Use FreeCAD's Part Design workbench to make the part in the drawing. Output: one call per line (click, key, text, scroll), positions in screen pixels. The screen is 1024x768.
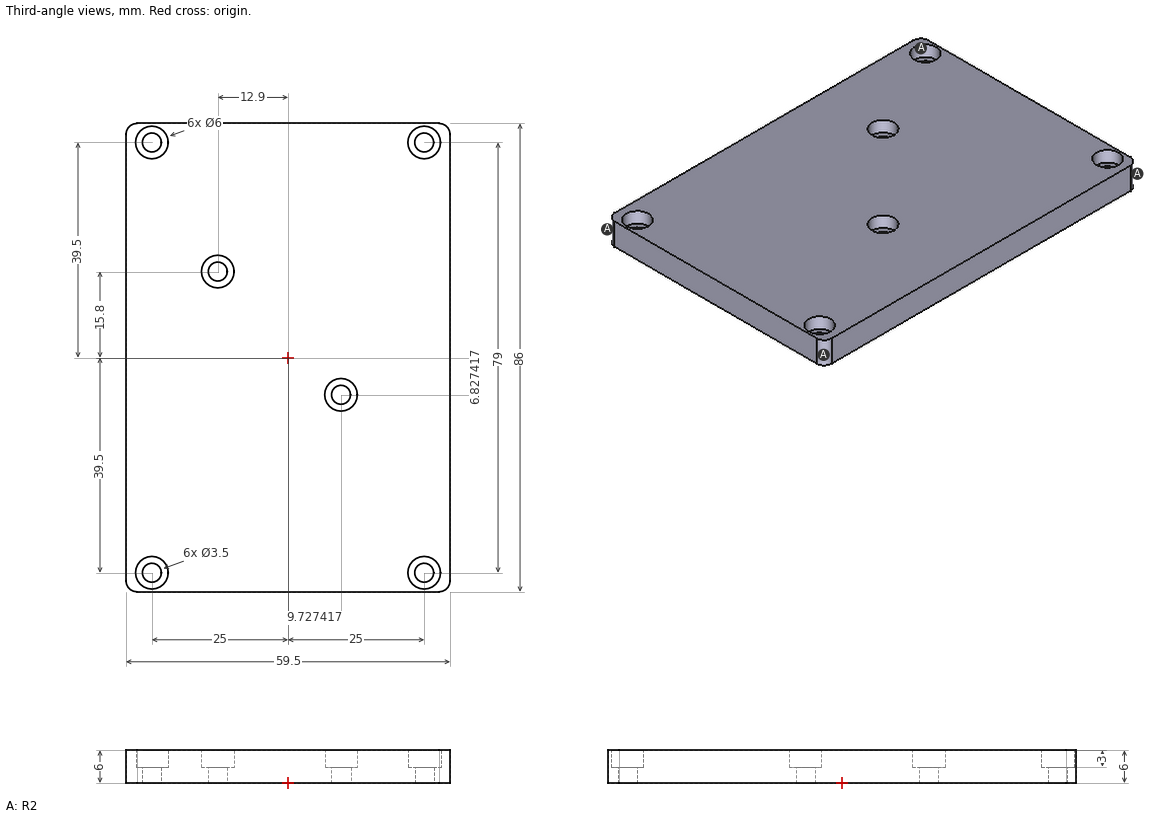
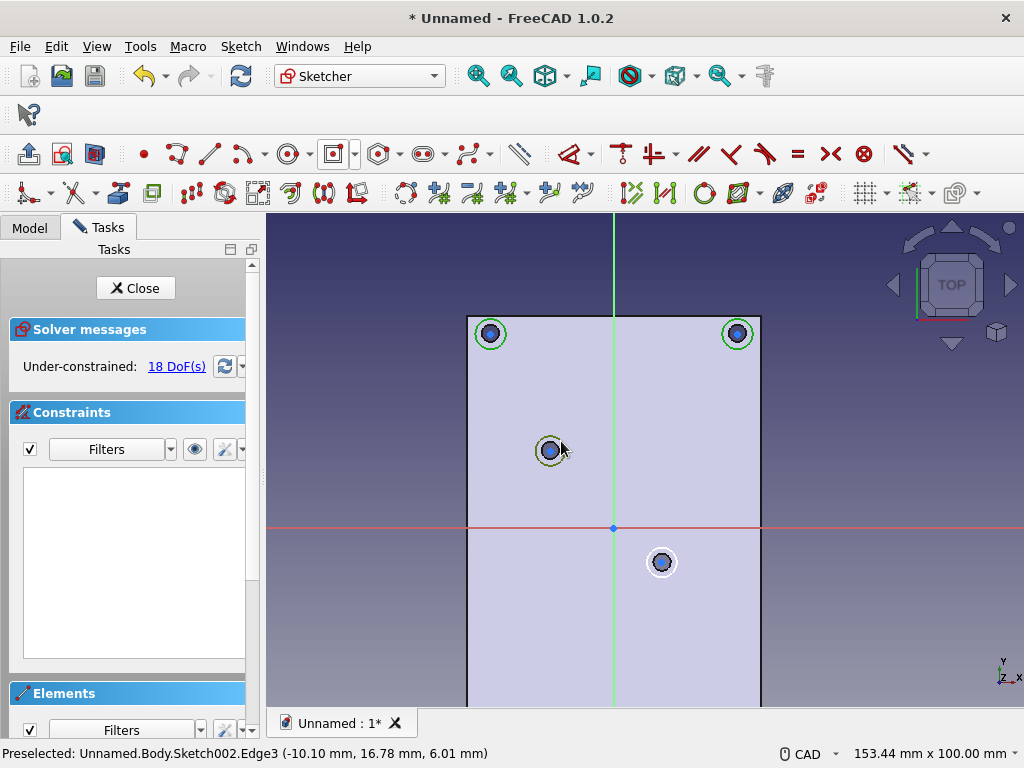
click(672, 552)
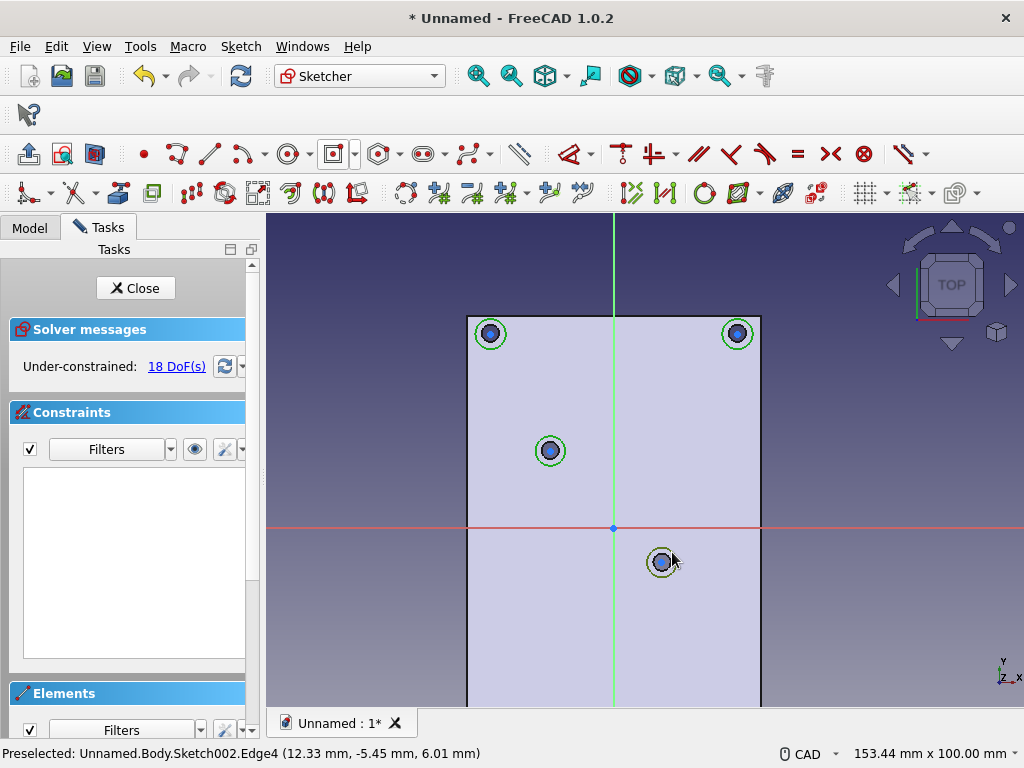
scroll(500, 321, down, 2)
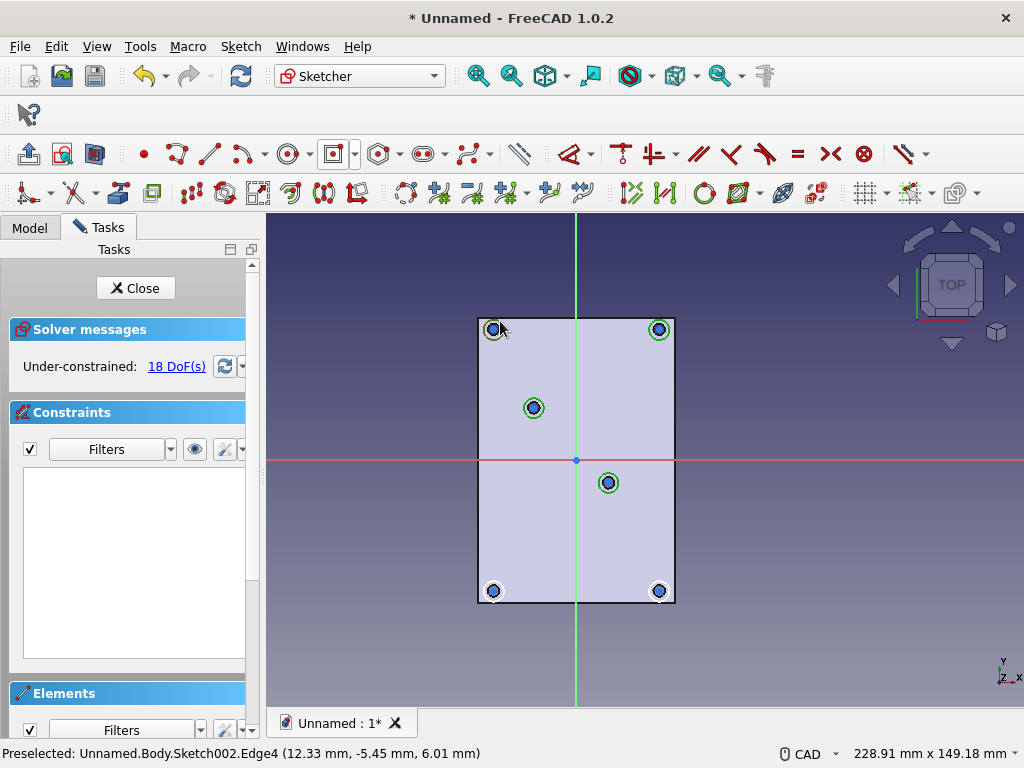
scroll(501, 584, up, 2)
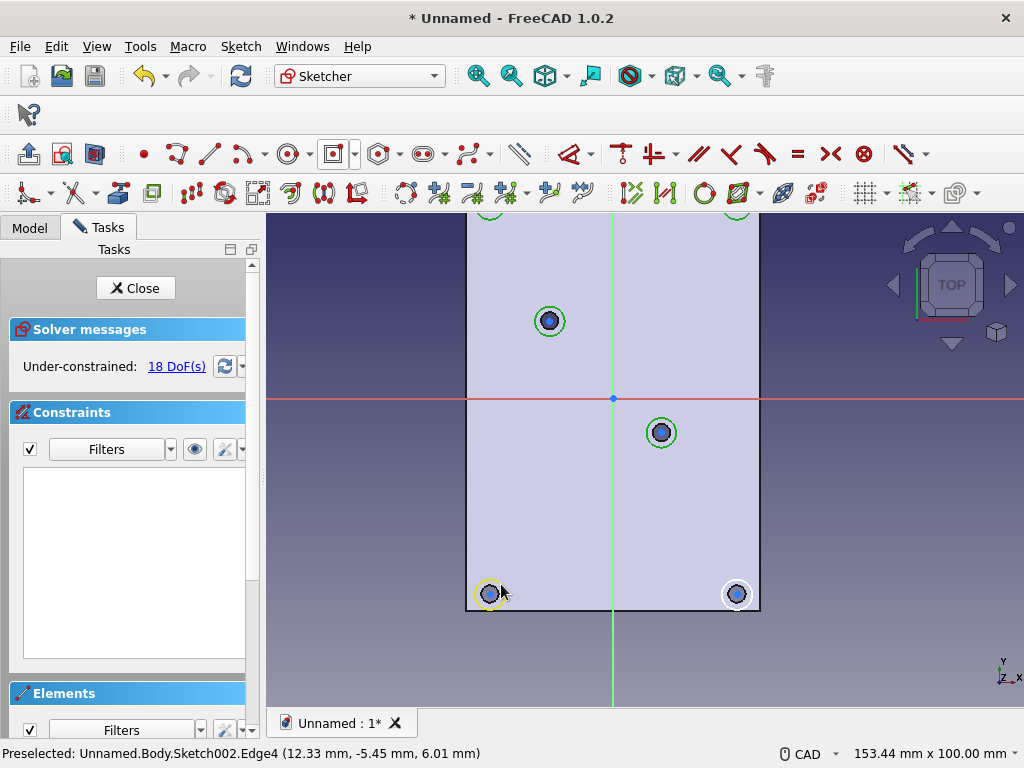
click(501, 584)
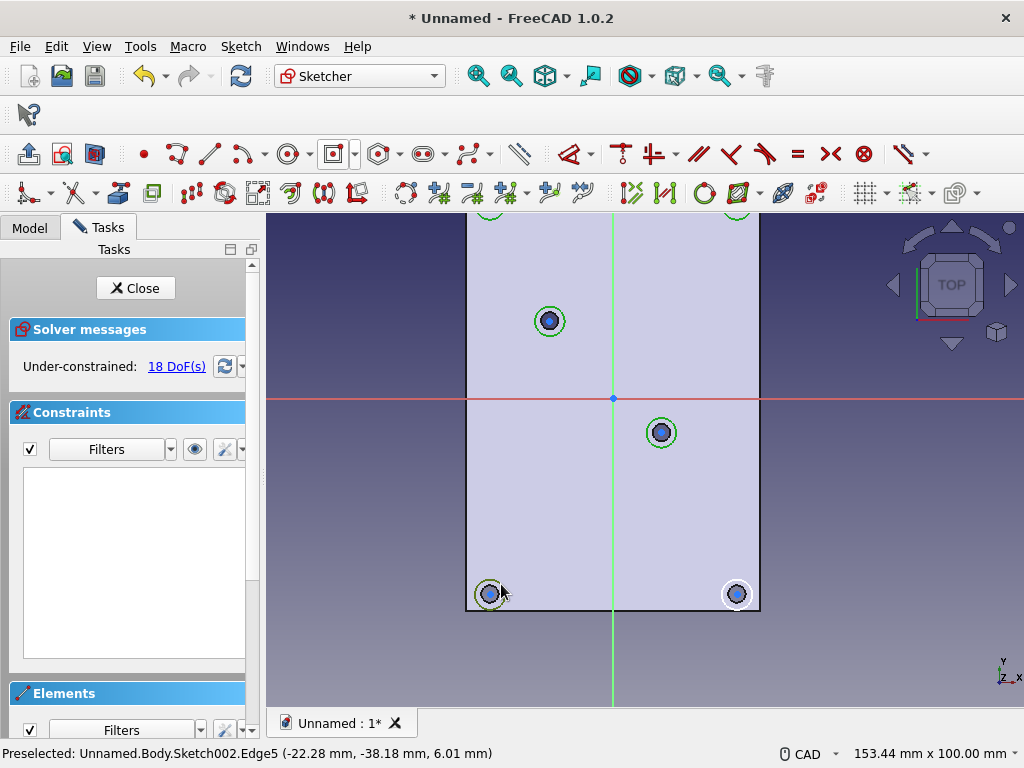
click(748, 584)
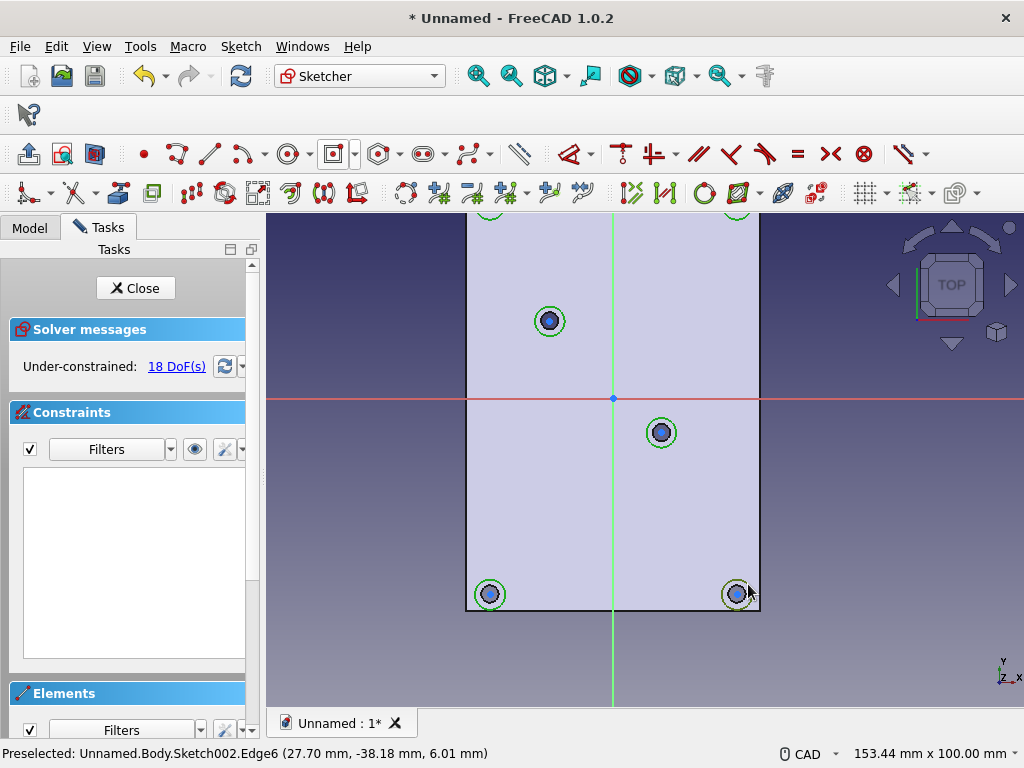
click(798, 154)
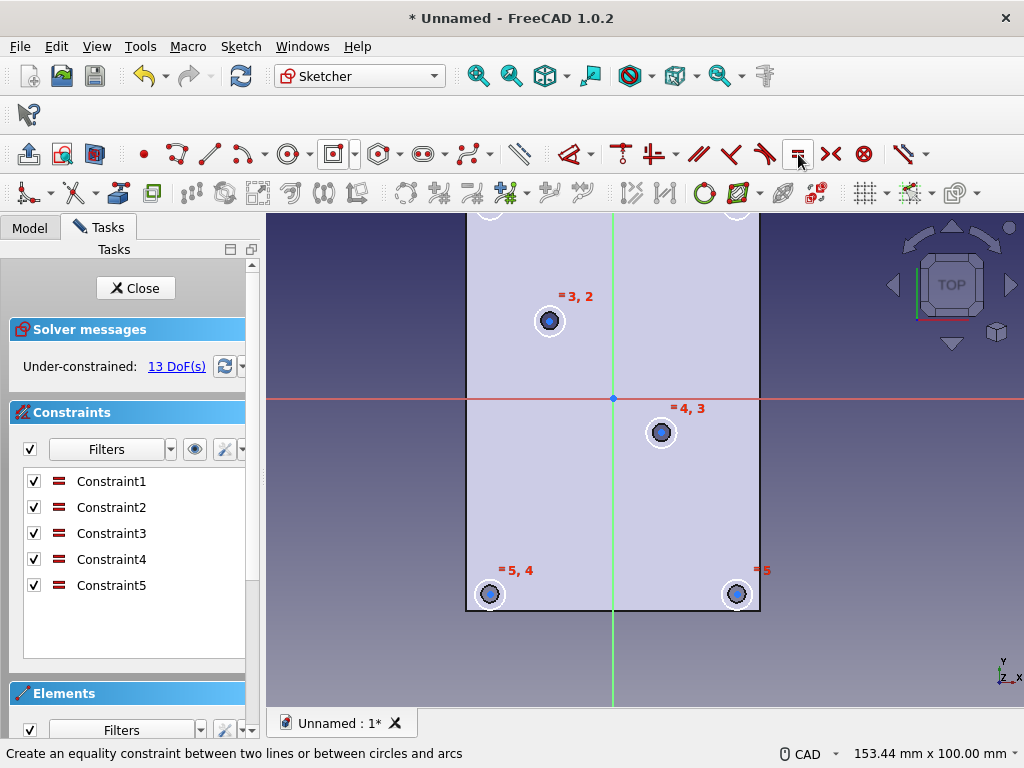
scroll(501, 584, down, 2)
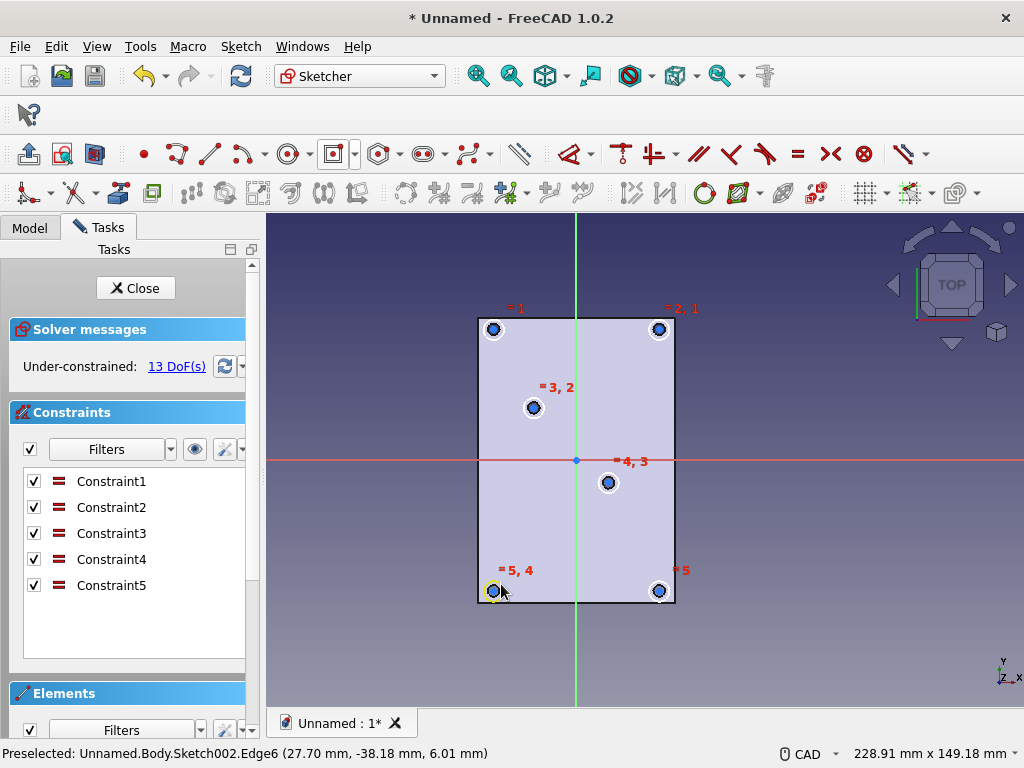
click(494, 330)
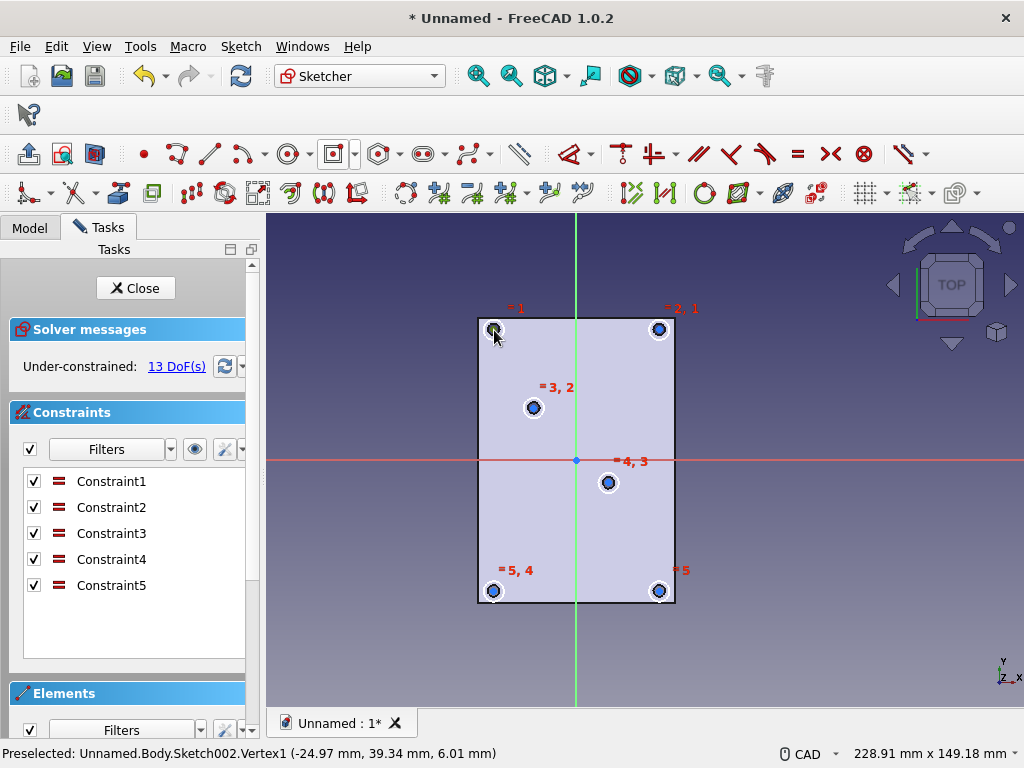
click(659, 330)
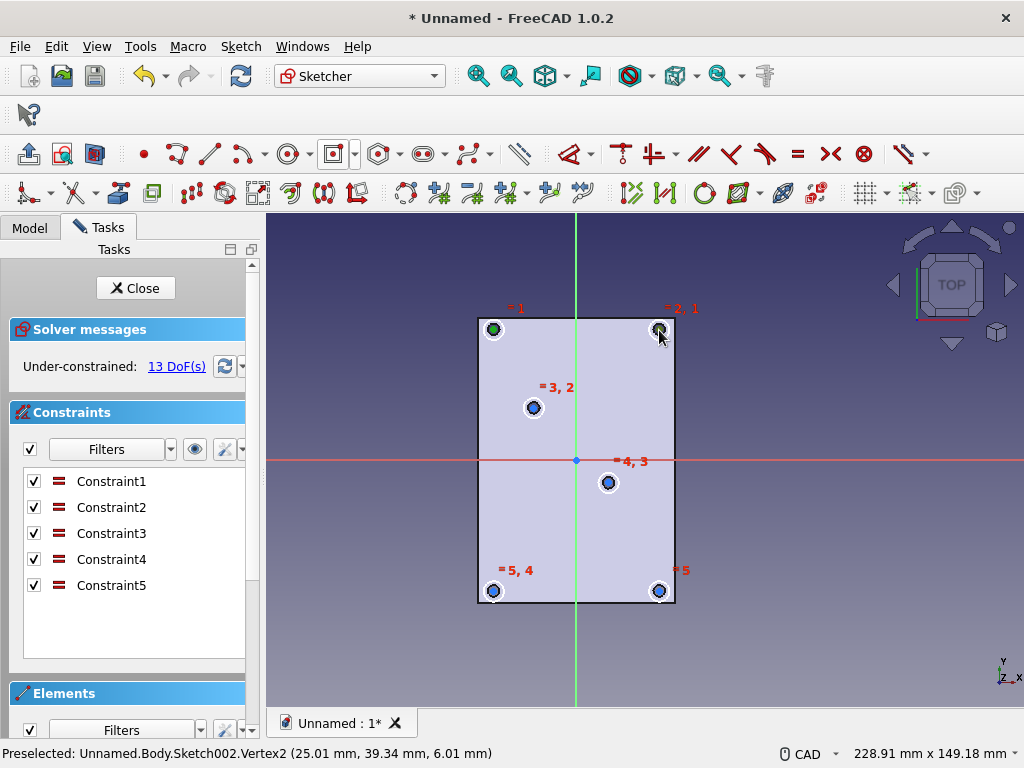
key(h)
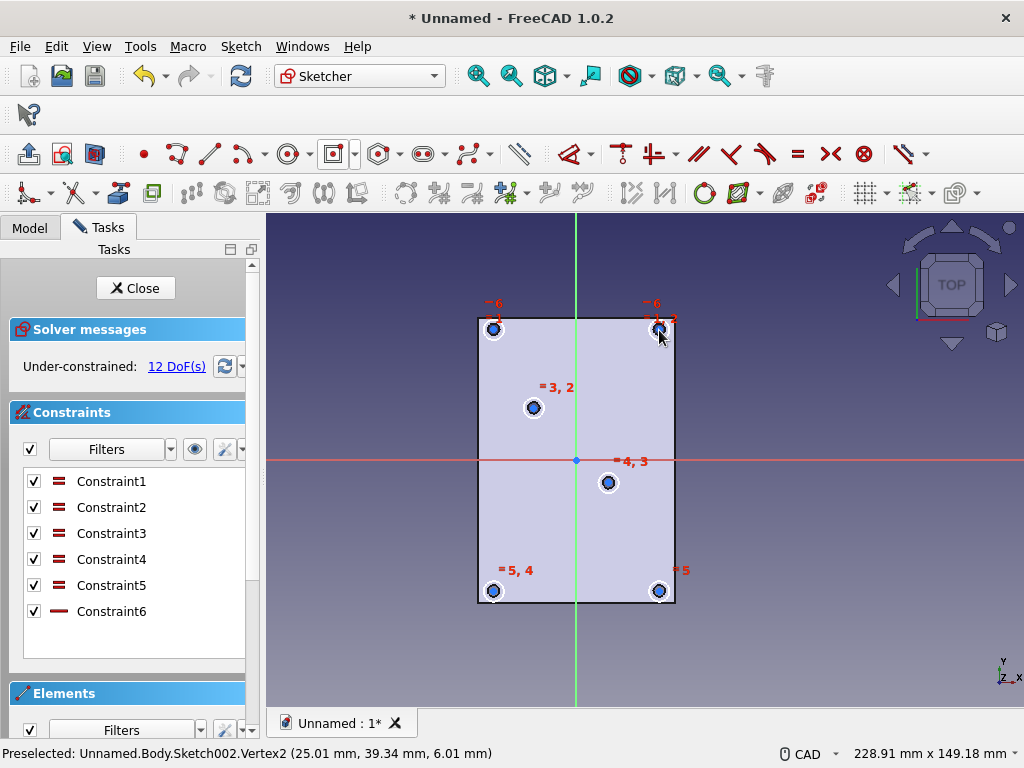
click(494, 330)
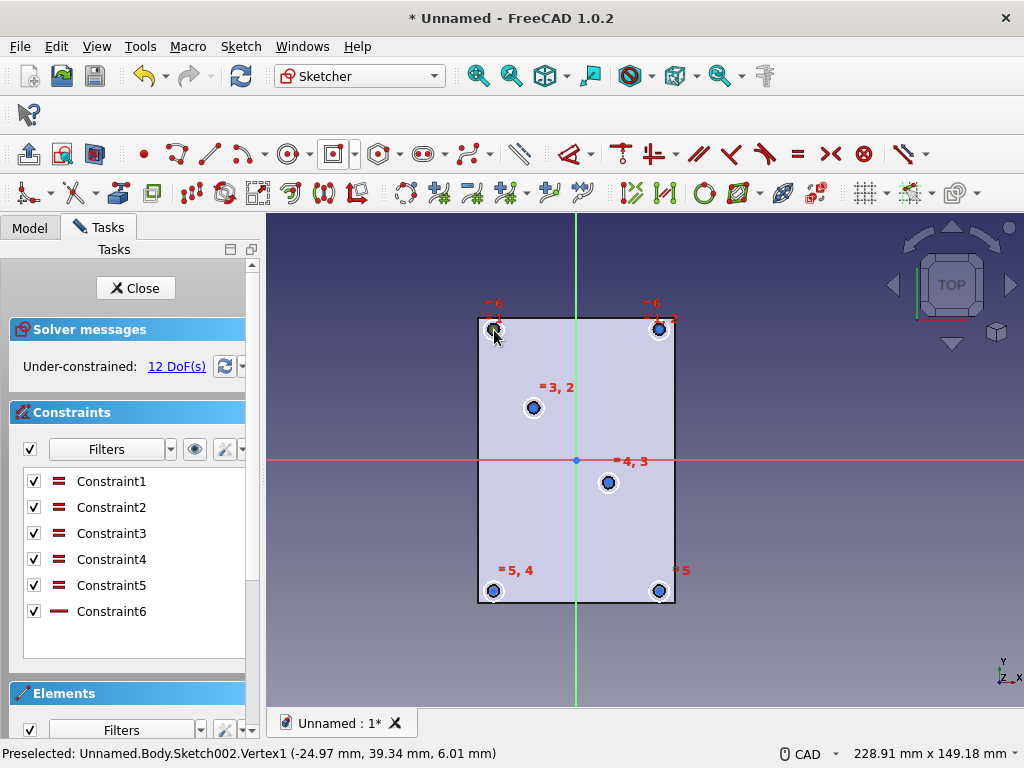
click(494, 591)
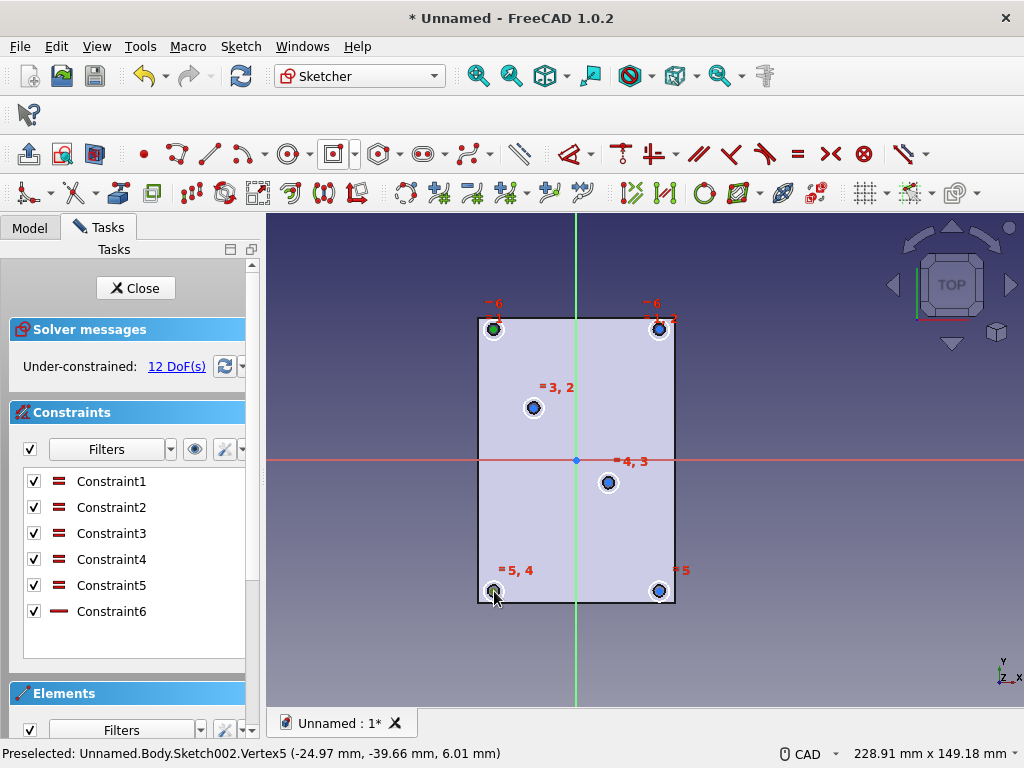
key(v)